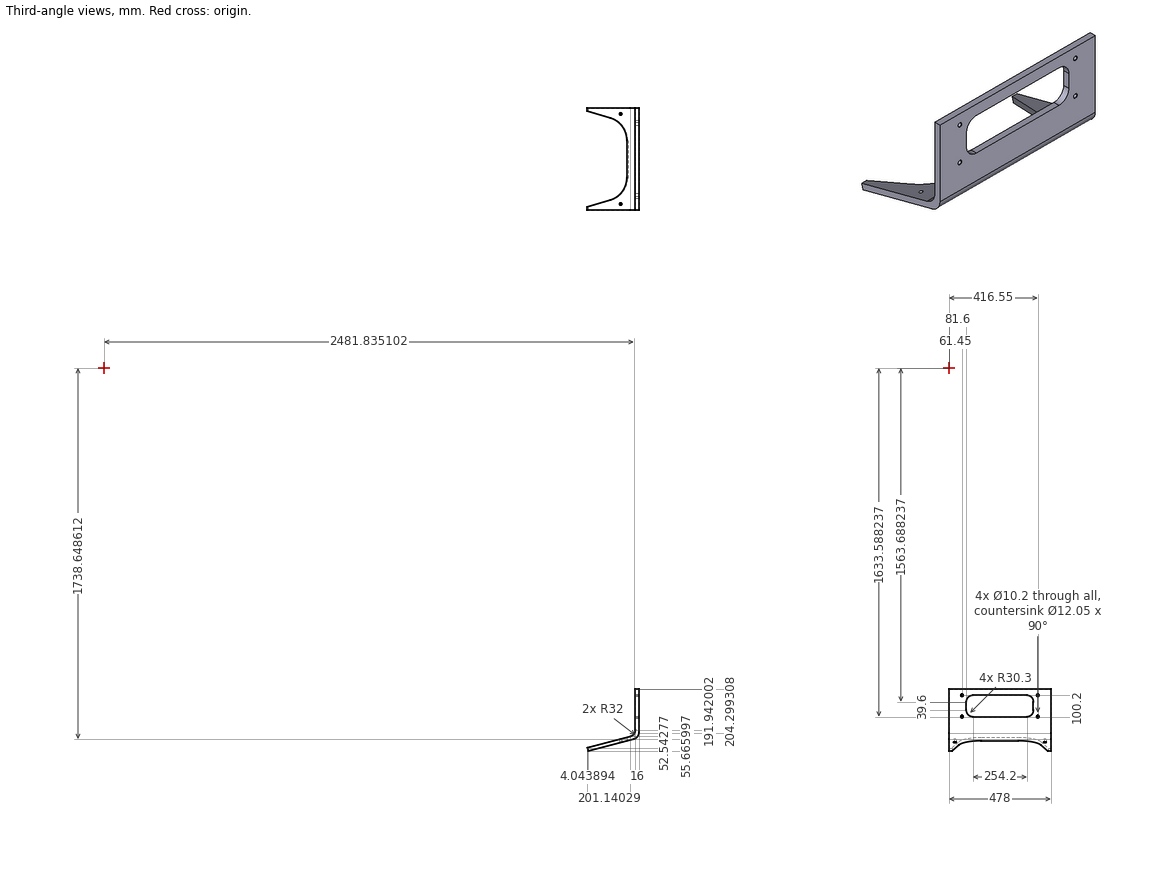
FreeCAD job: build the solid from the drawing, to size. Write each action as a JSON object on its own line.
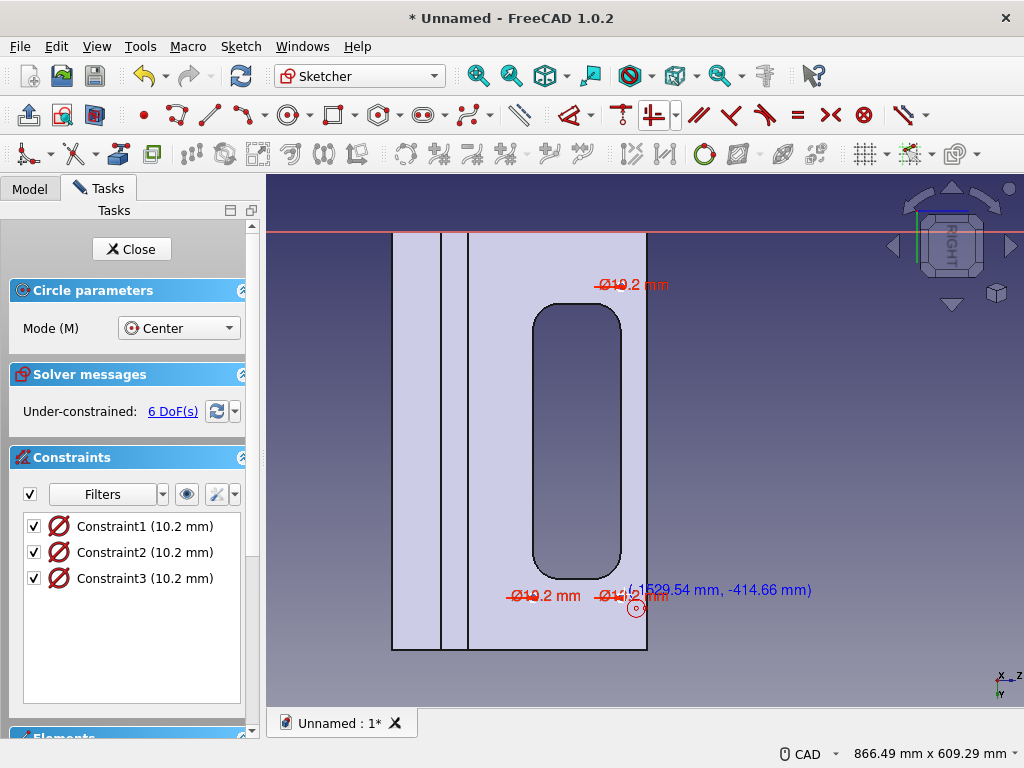
{"action": "scroll", "coordinate": [533, 286], "scroll_direction": "up", "scroll_amount": 9}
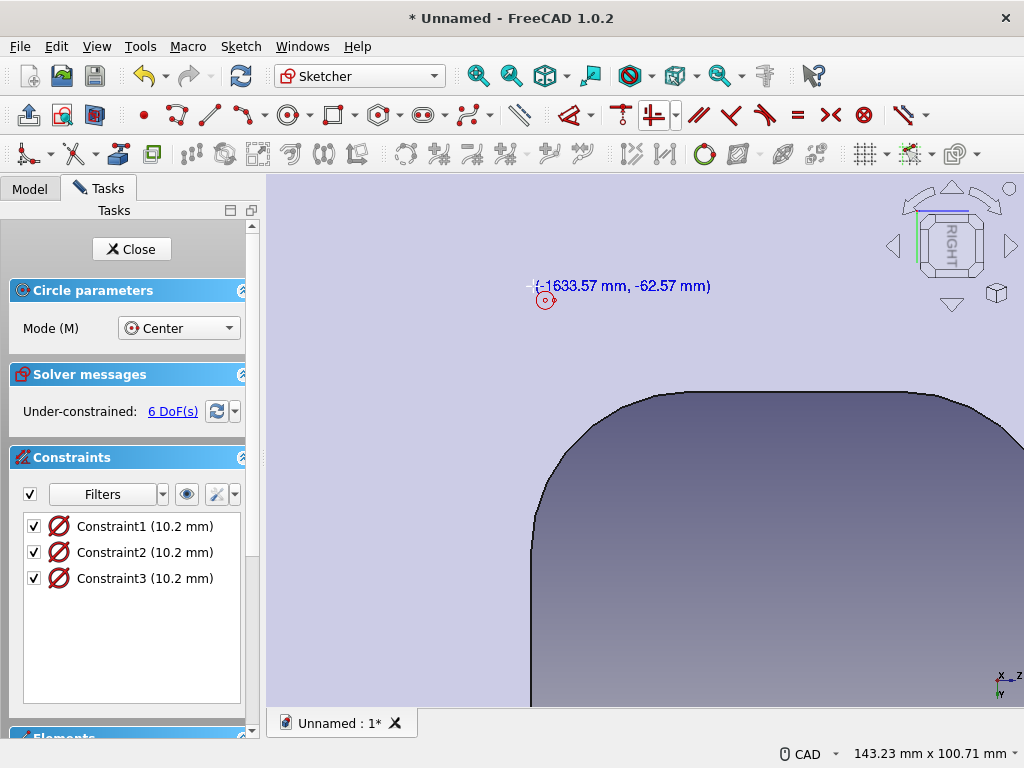
{"action": "scroll", "coordinate": [533, 285], "scroll_direction": "down", "scroll_amount": 9}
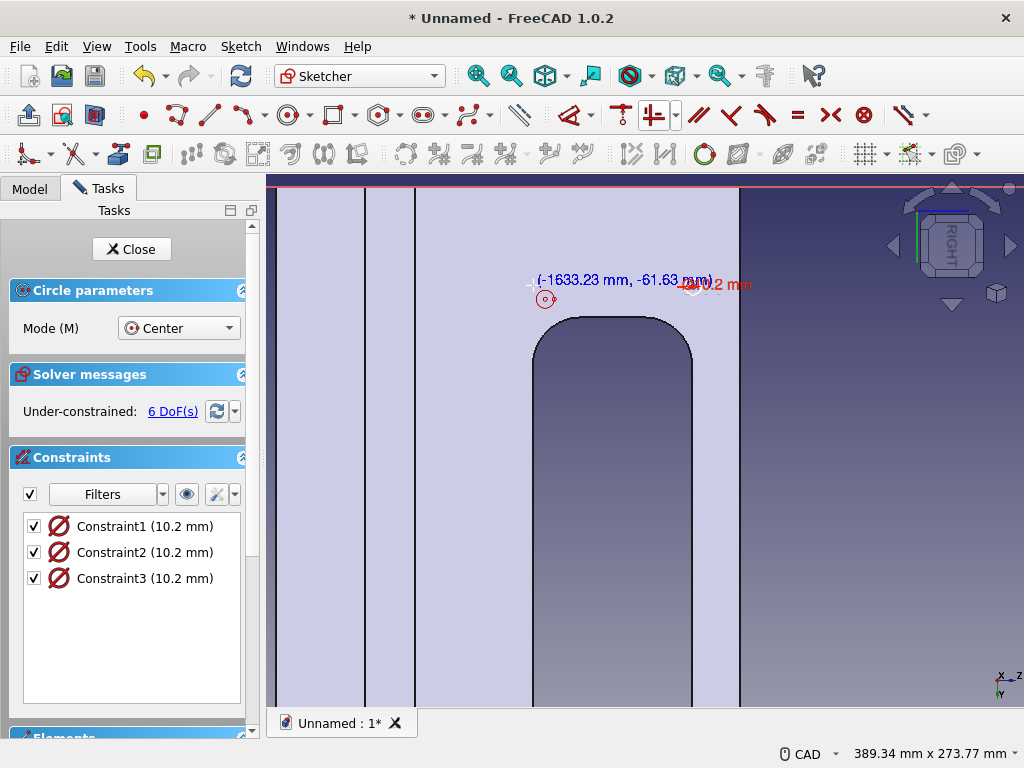
{"action": "left_click", "coordinate": [533, 285]}
{"action": "mouse_move", "coordinate": [536, 282]}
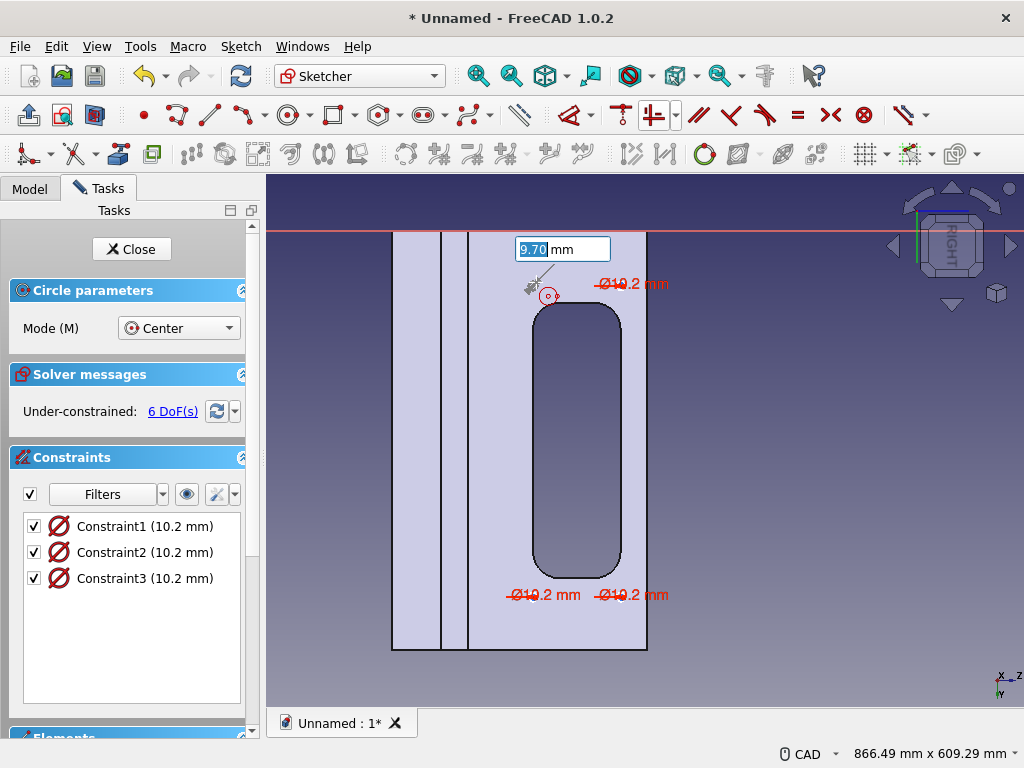
{"action": "type", "text": "10.2"}
{"action": "key", "text": "Return"}
{"action": "key", "text": "Escape"}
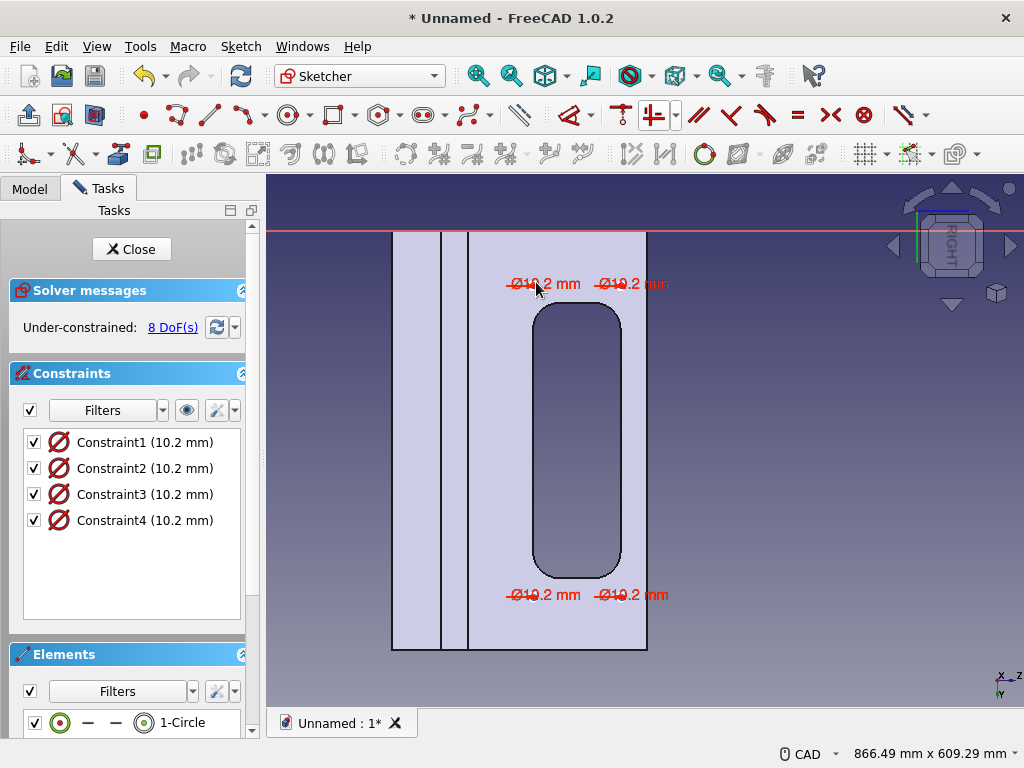
{"action": "left_click", "coordinate": [568, 116]}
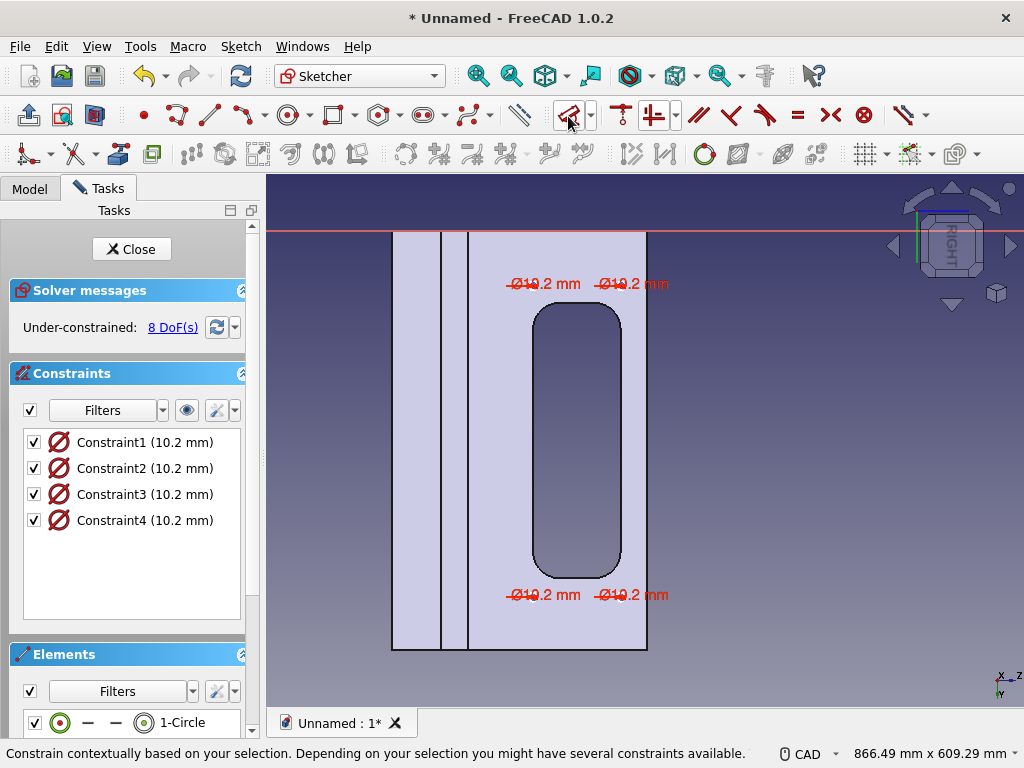
{"action": "left_click", "coordinate": [621, 286]}
{"action": "left_click", "coordinate": [587, 259]}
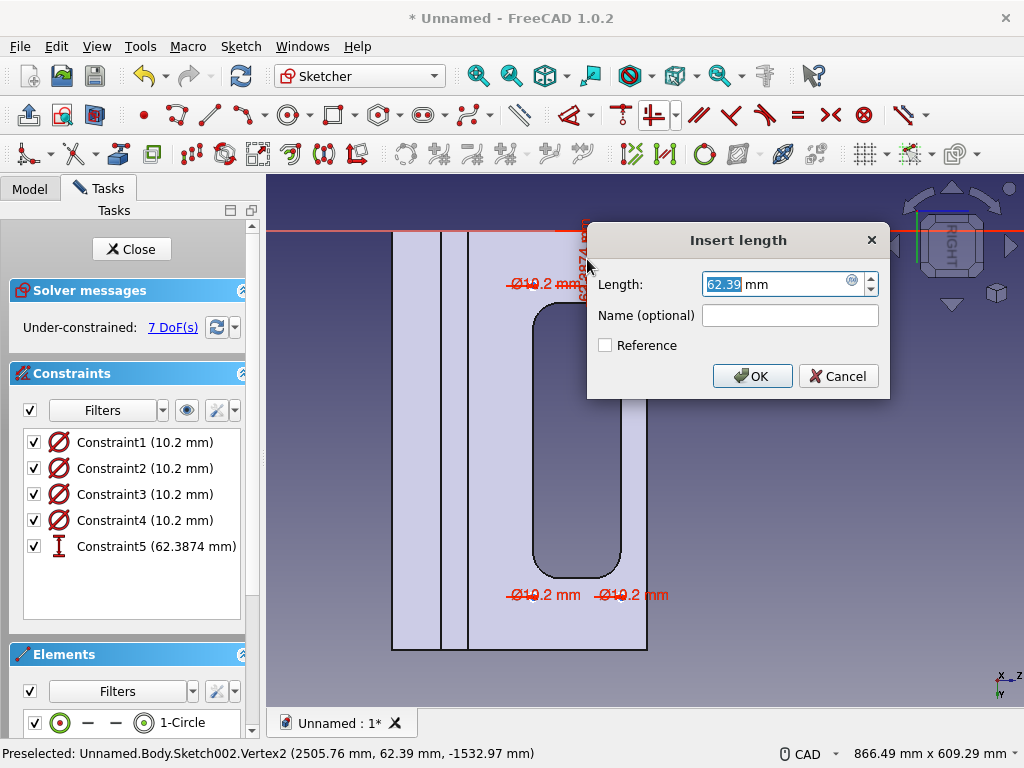
{"action": "type", "text": "61.45"}
{"action": "key", "text": "Return"}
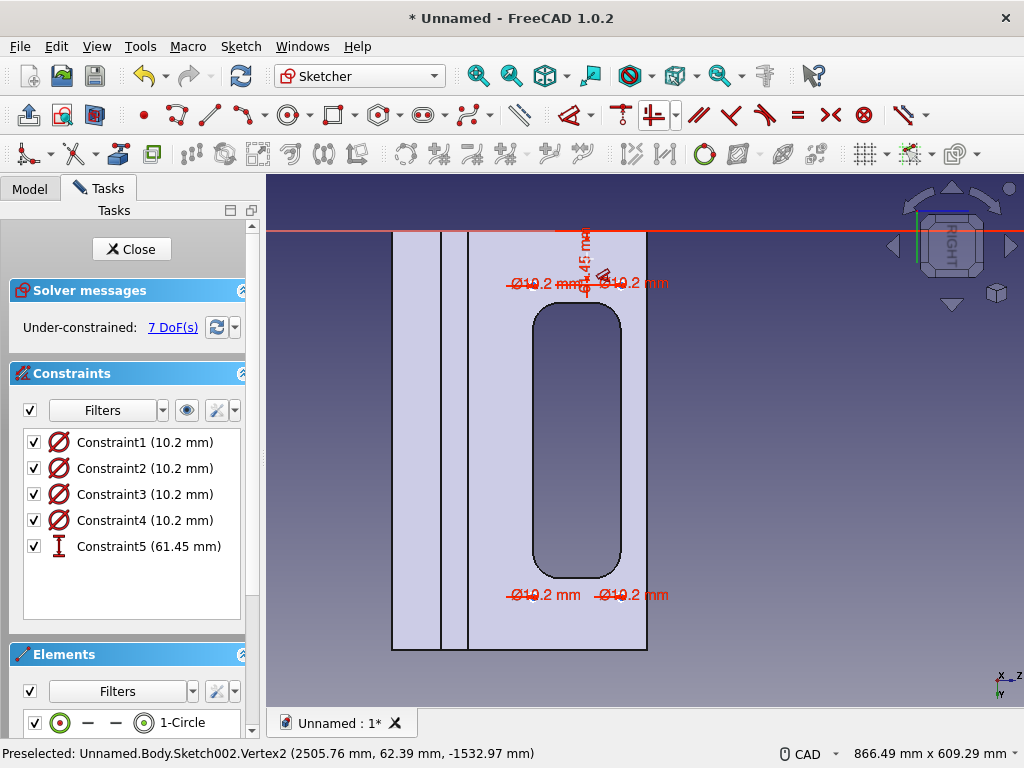
{"action": "left_click", "coordinate": [533, 286]}
{"action": "left_click", "coordinate": [499, 259]}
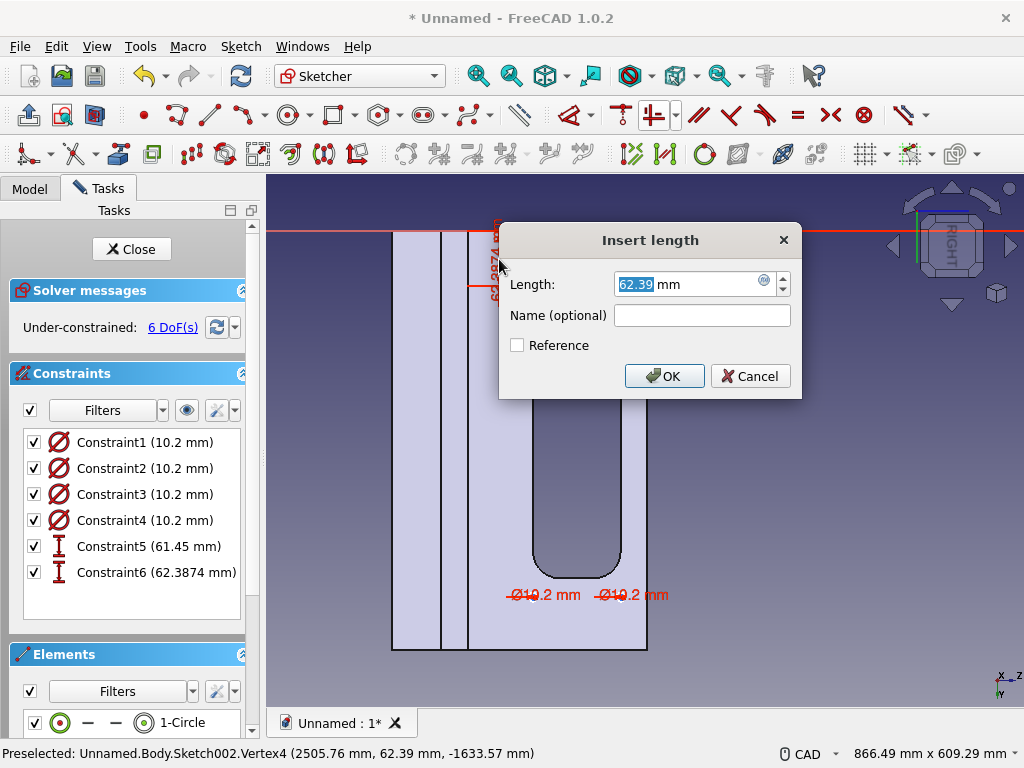
{"action": "type", "text": "61.45"}
{"action": "key", "text": "Return"}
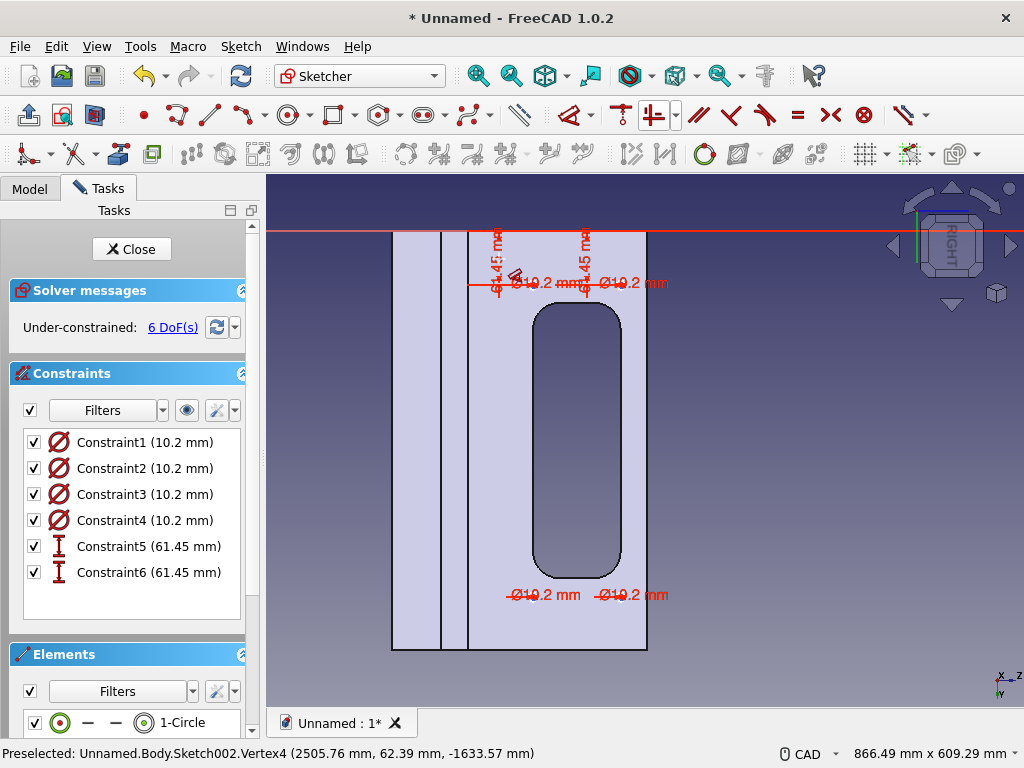
{"action": "left_click", "coordinate": [533, 597]}
{"action": "left_click", "coordinate": [499, 414]}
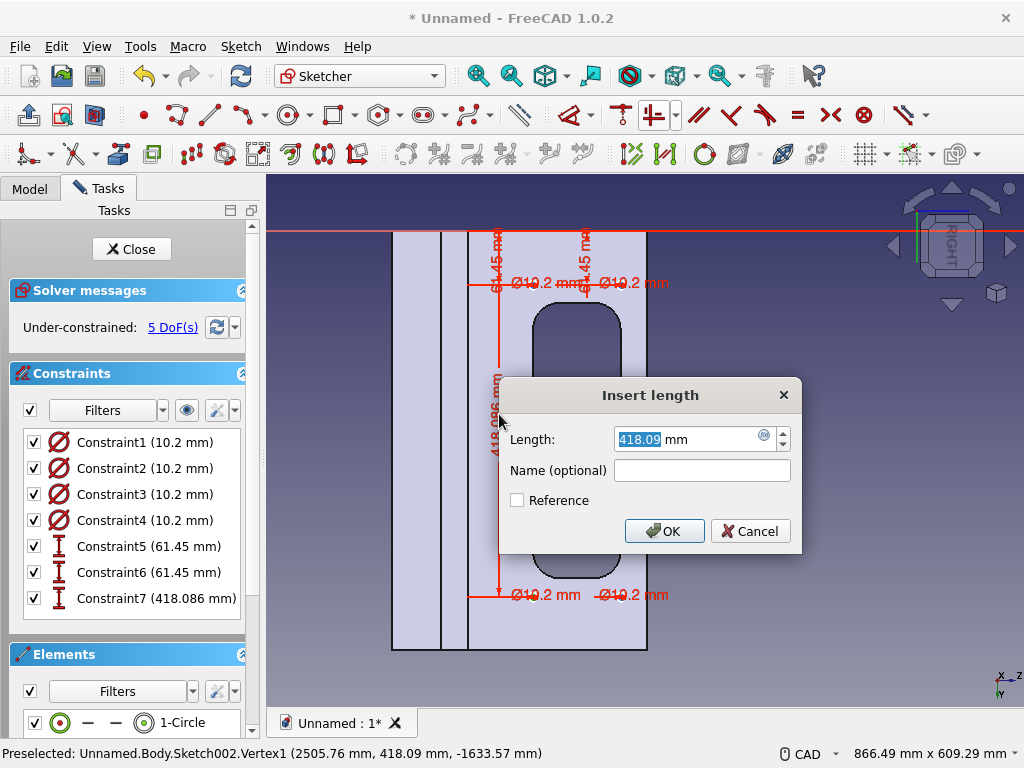
{"action": "type", "text": "416.55"}
{"action": "key", "text": "Return"}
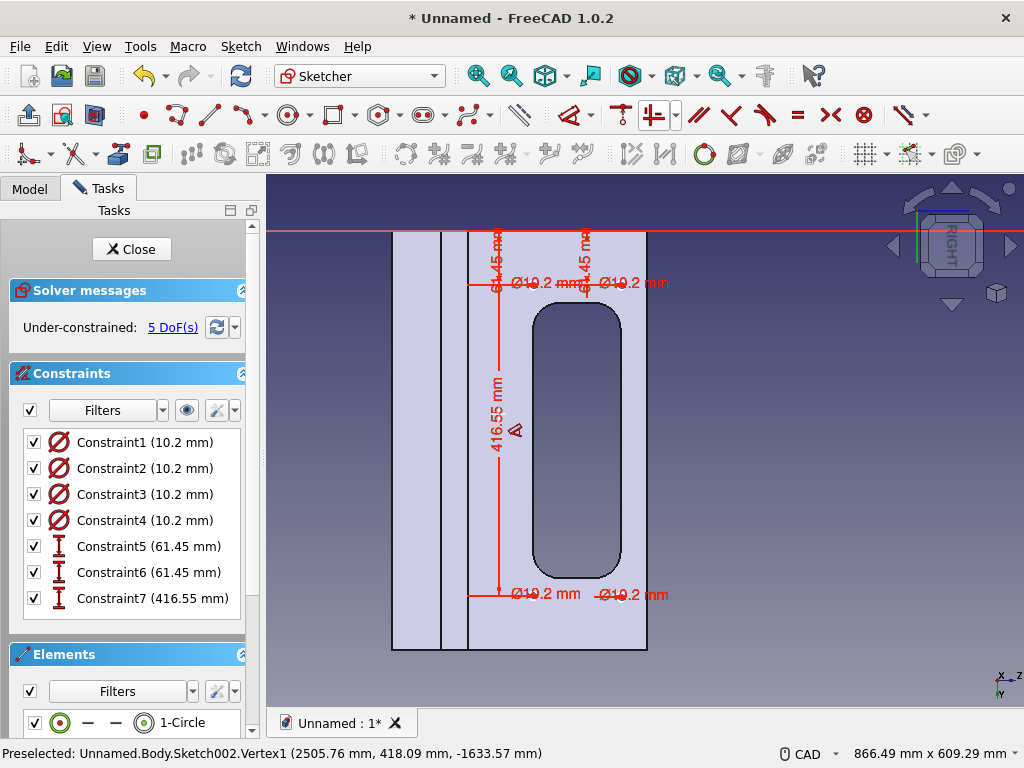
{"action": "left_click", "coordinate": [621, 597]}
{"action": "left_click", "coordinate": [587, 414]}